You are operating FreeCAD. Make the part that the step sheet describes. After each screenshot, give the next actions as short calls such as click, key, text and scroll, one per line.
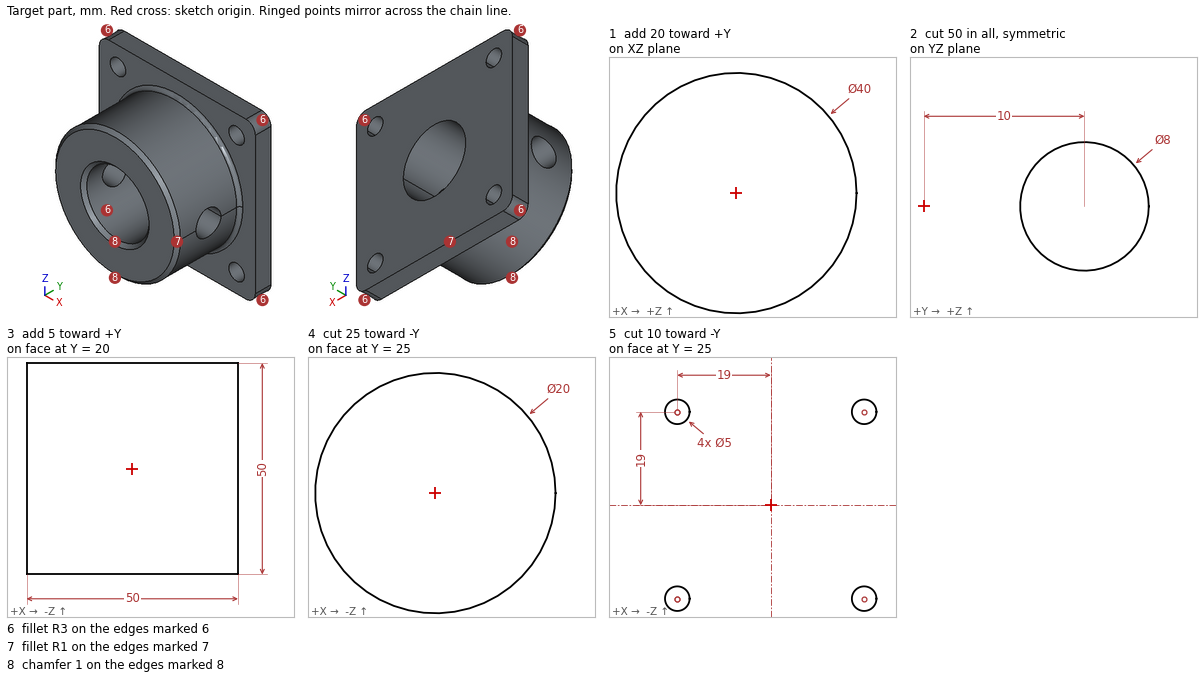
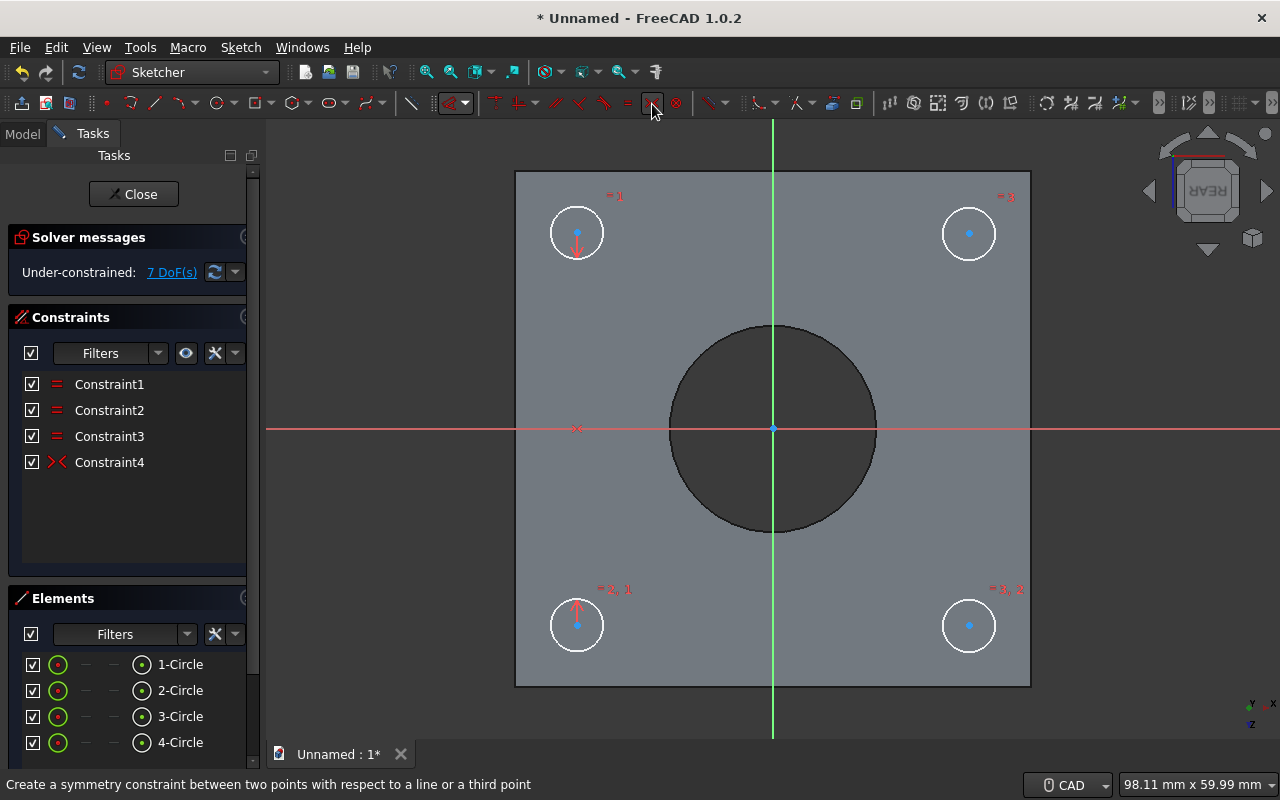
click(577, 625)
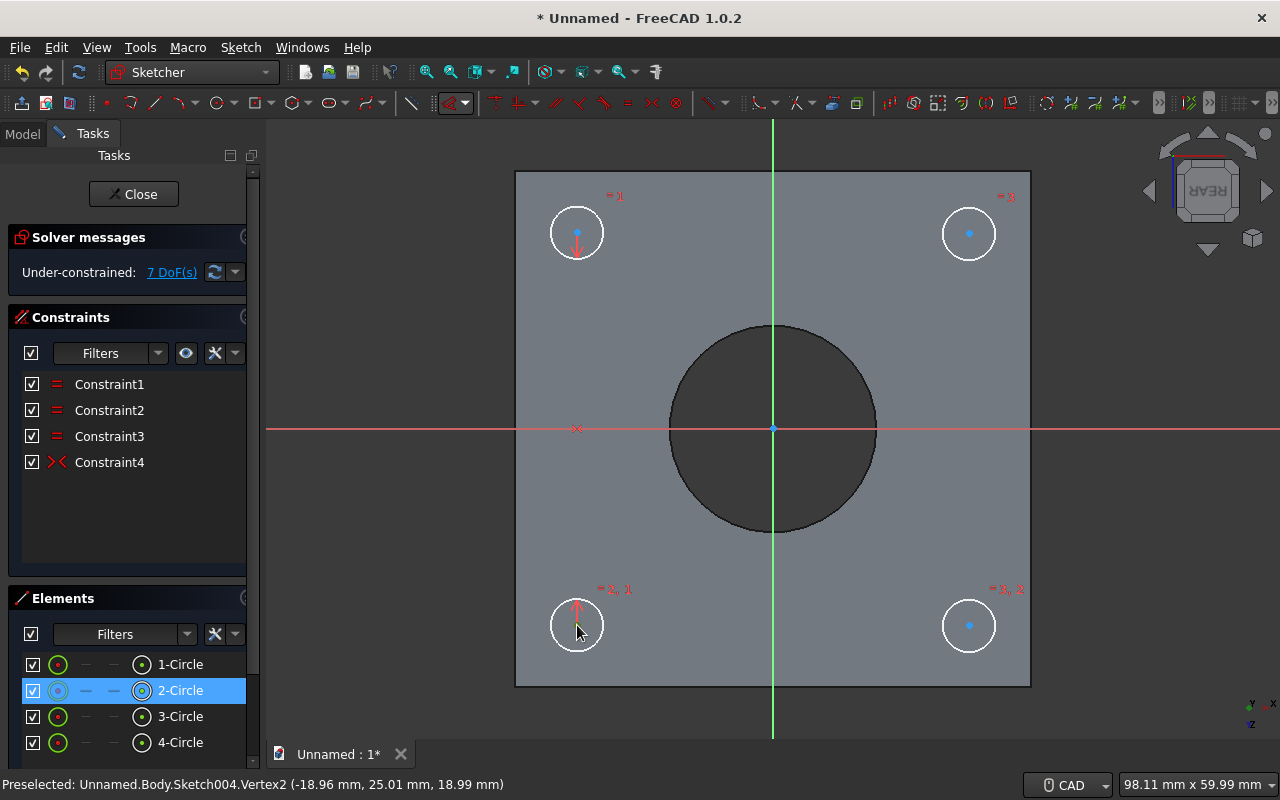
click(969, 626)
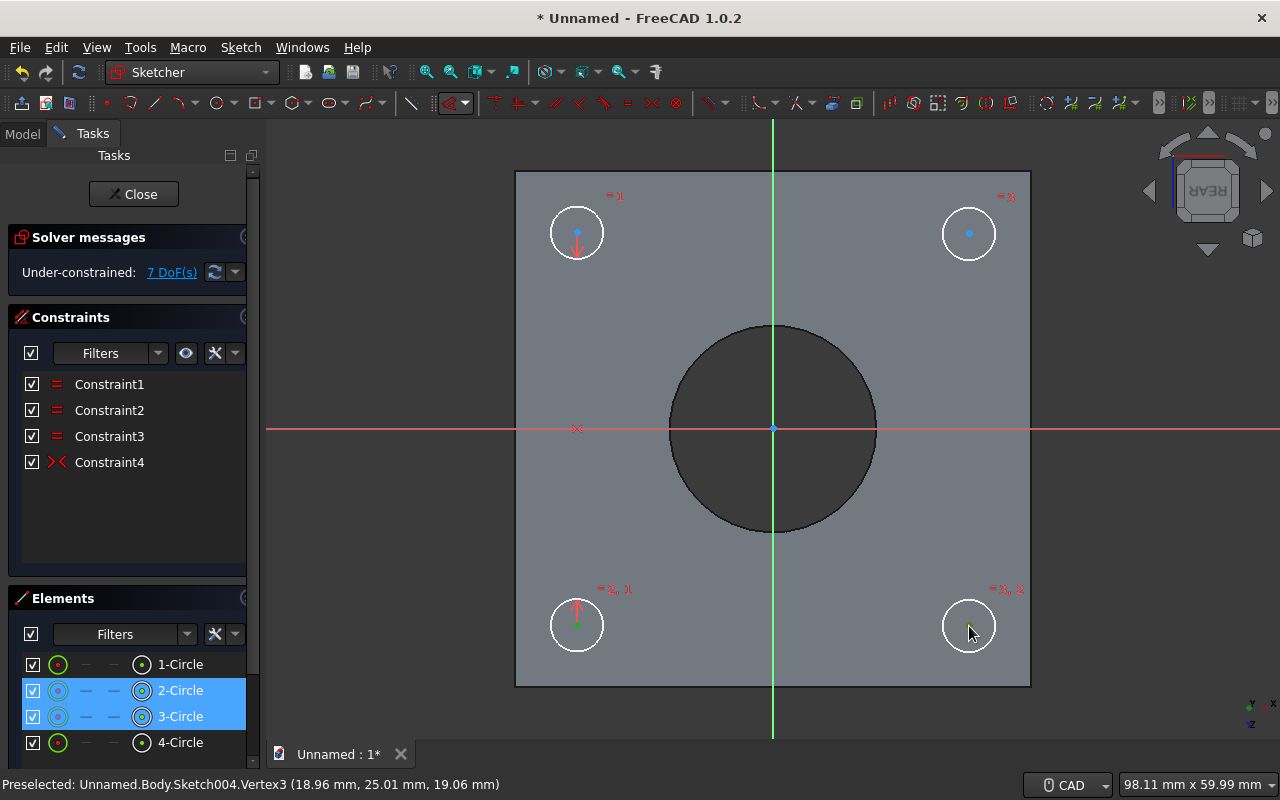
click(773, 671)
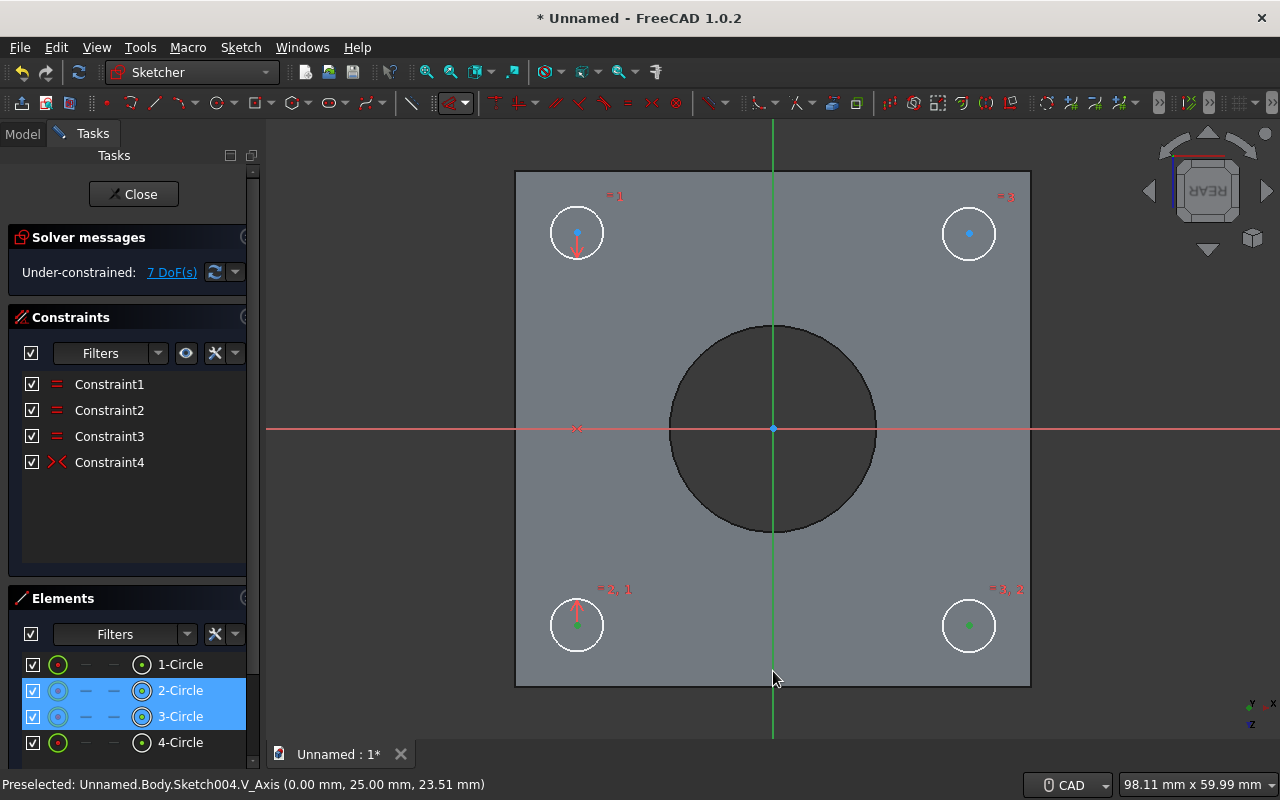
click(652, 104)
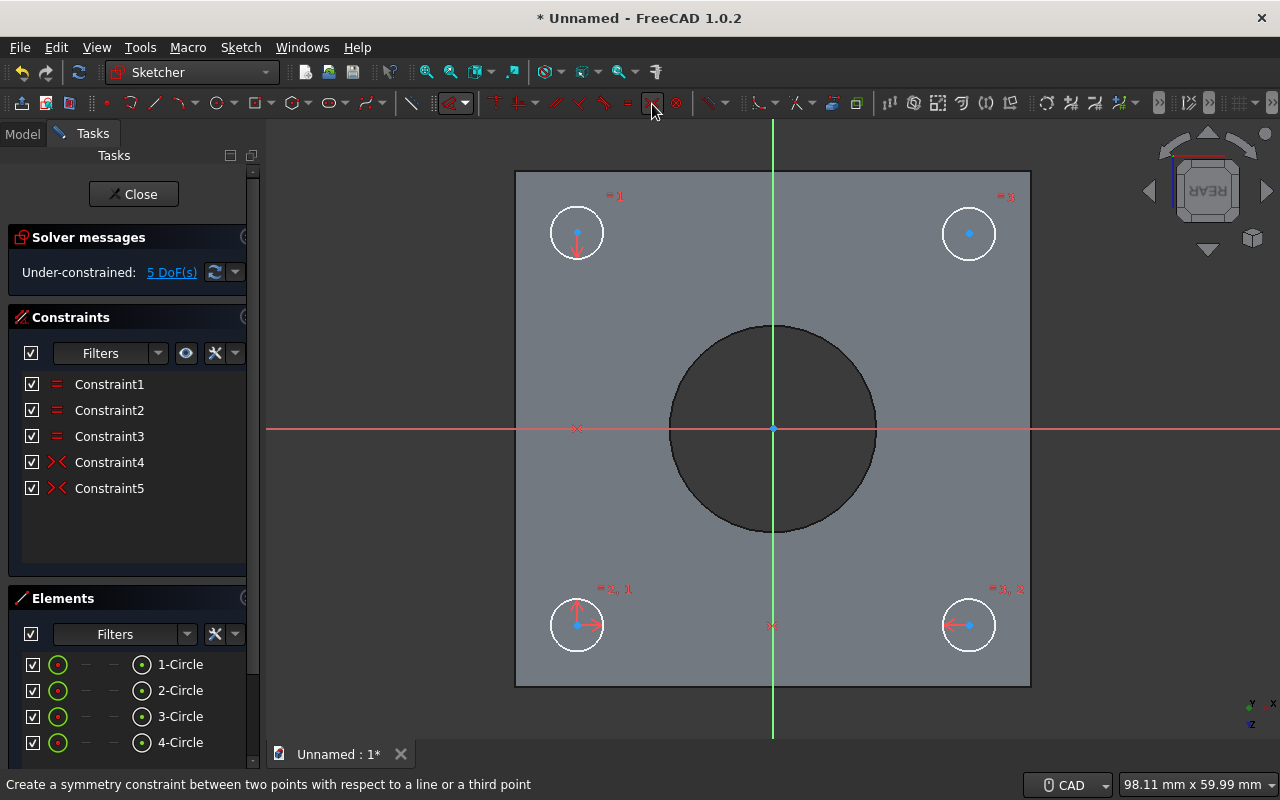
click(577, 233)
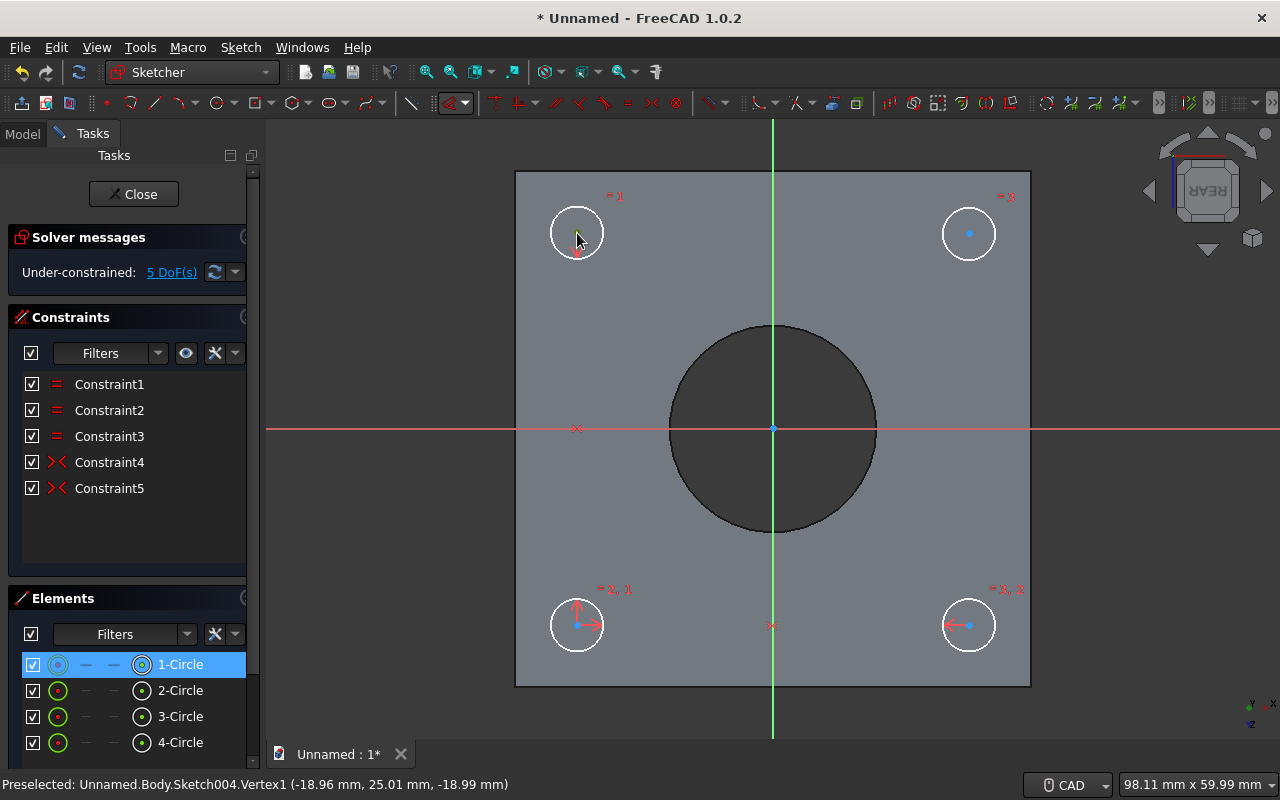
click(969, 234)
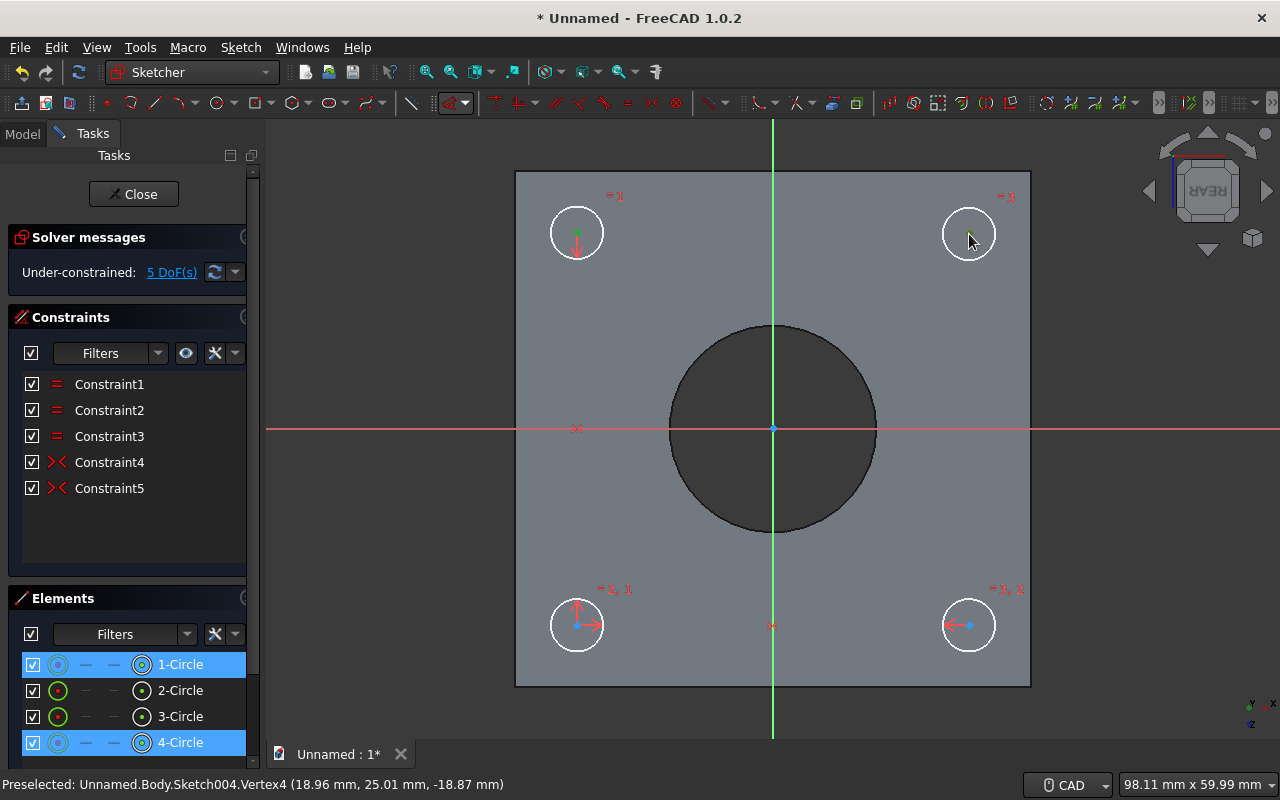
click(773, 671)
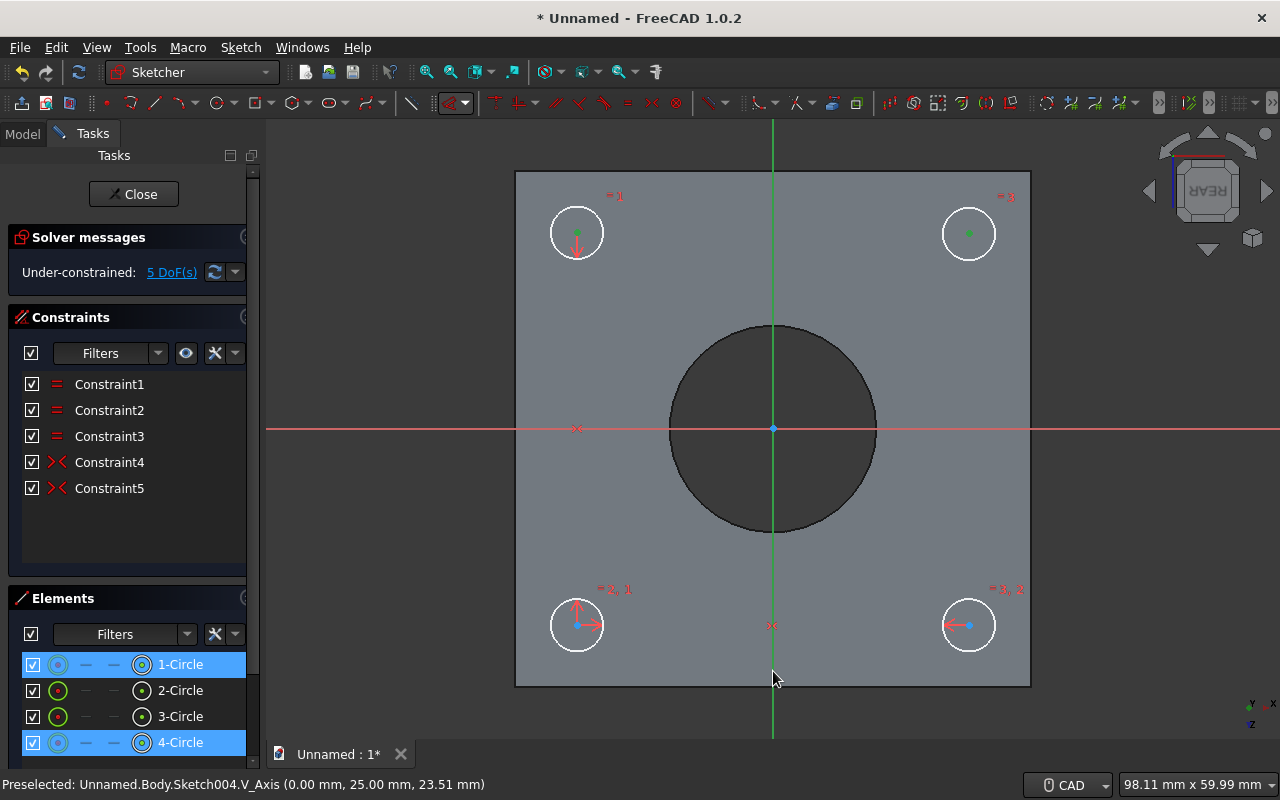
key(s)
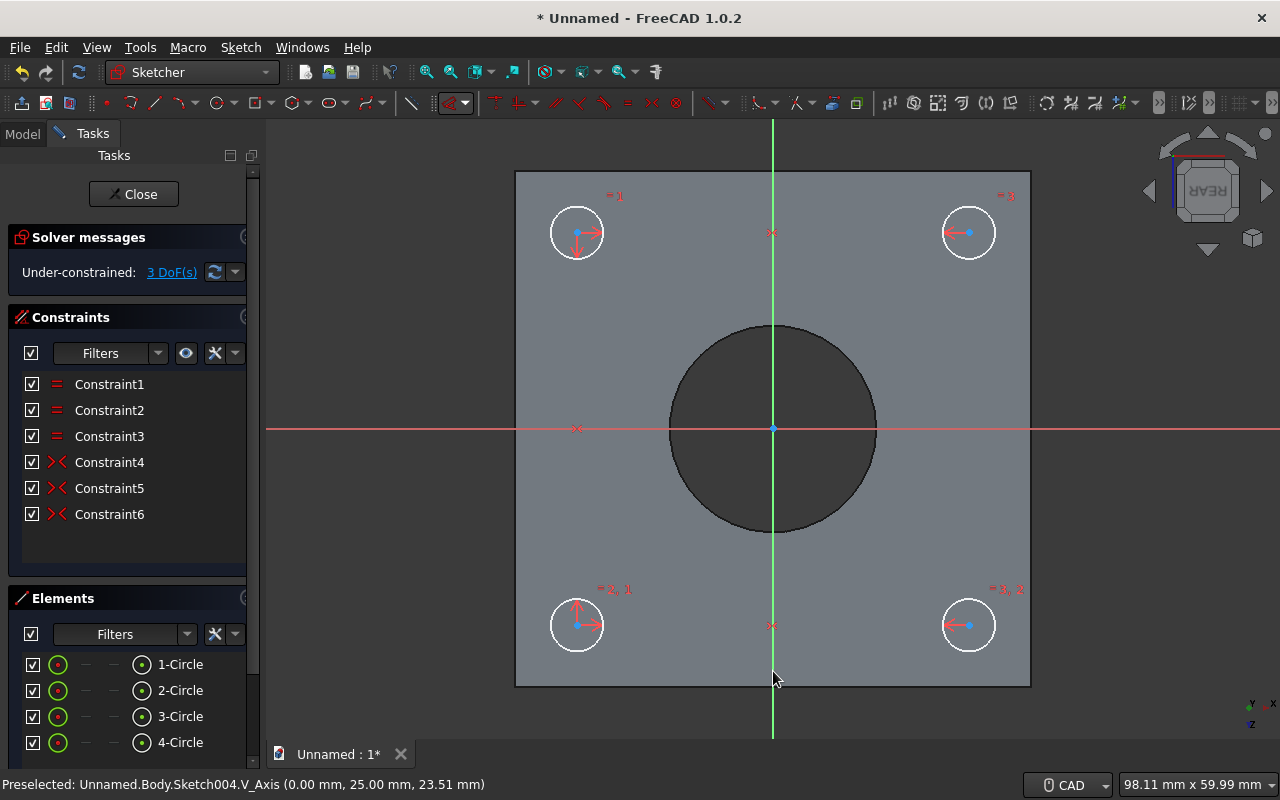
click(595, 214)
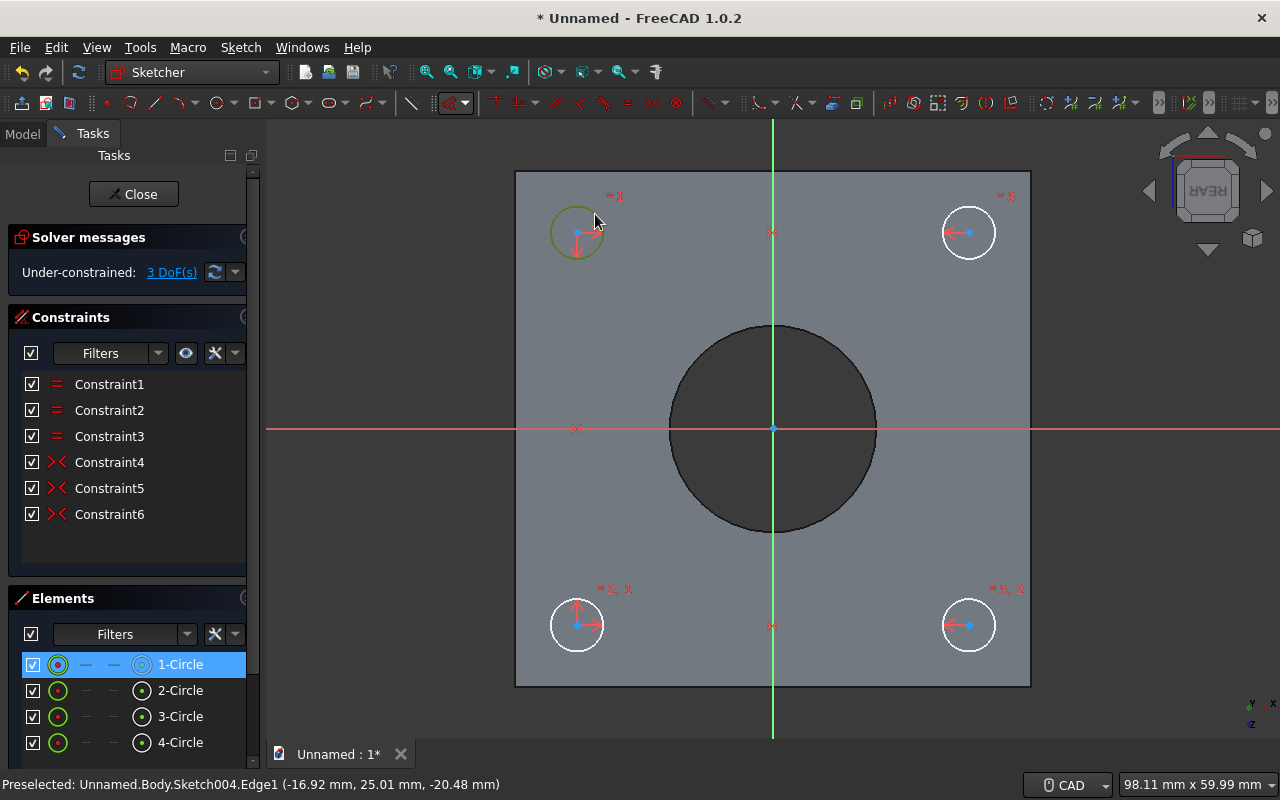
click(468, 104)